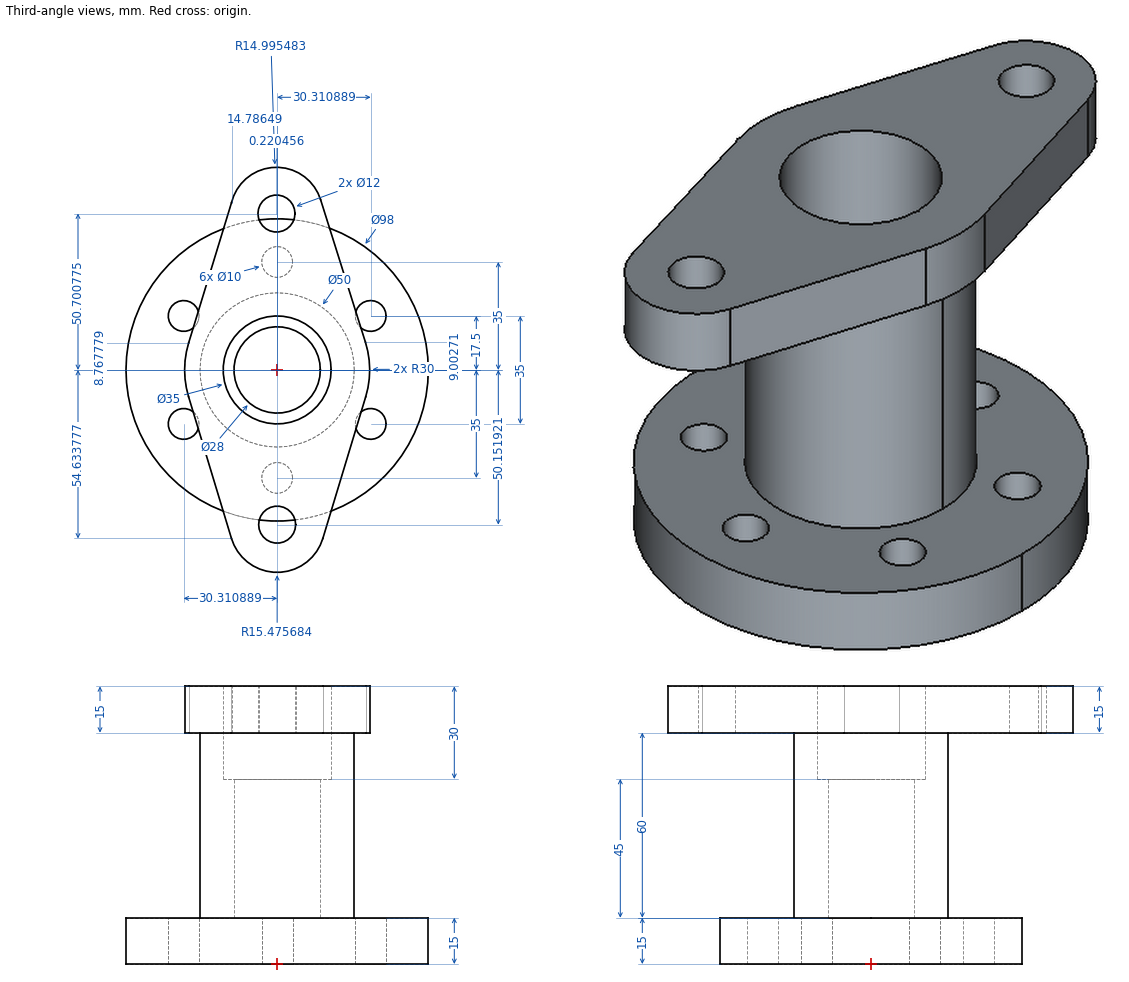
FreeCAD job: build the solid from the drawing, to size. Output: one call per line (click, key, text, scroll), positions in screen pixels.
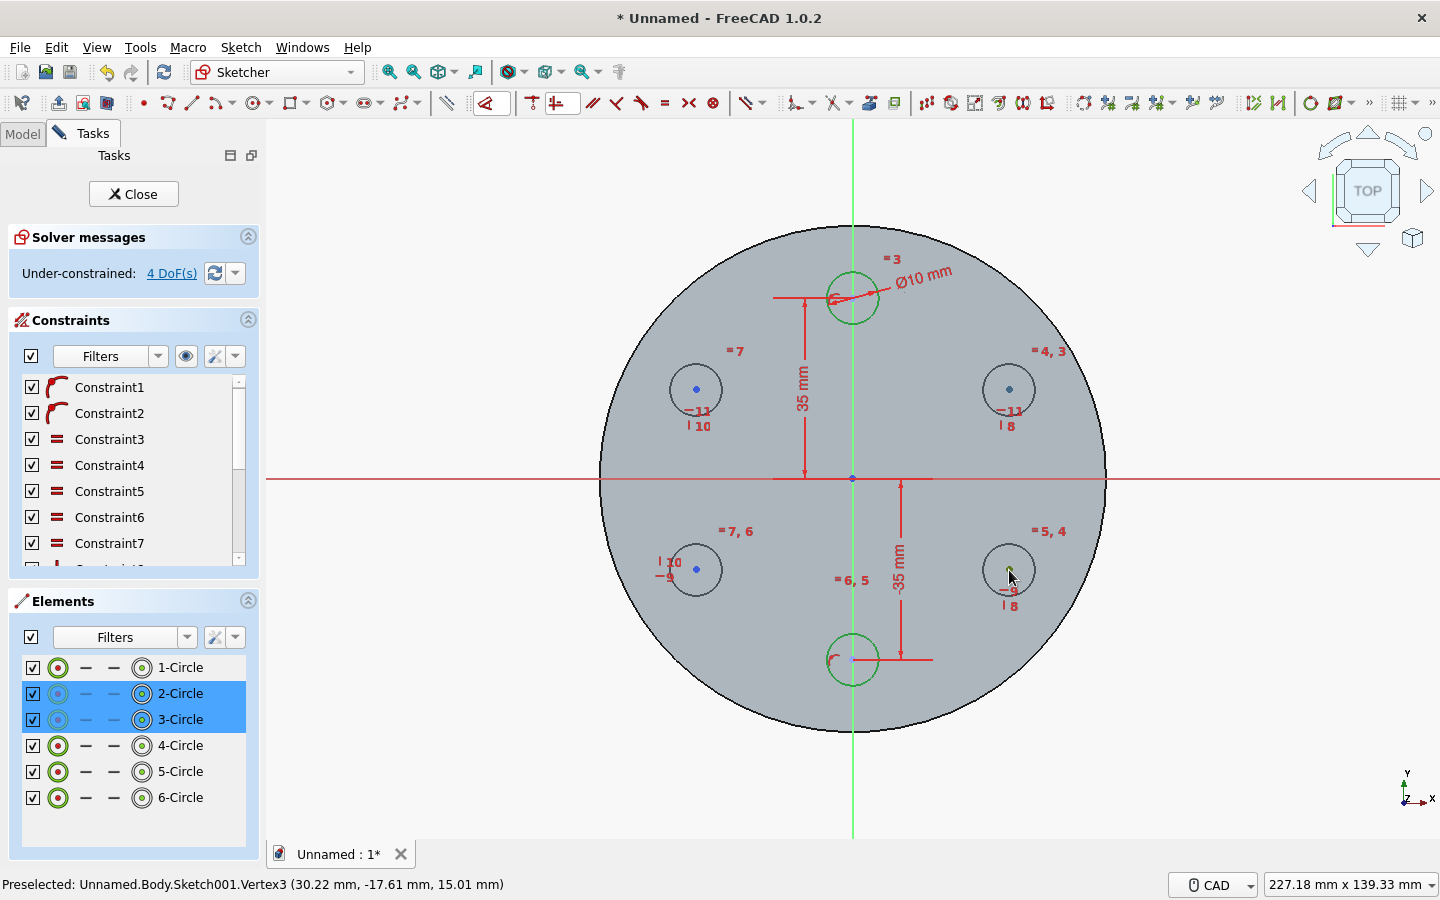
key(i)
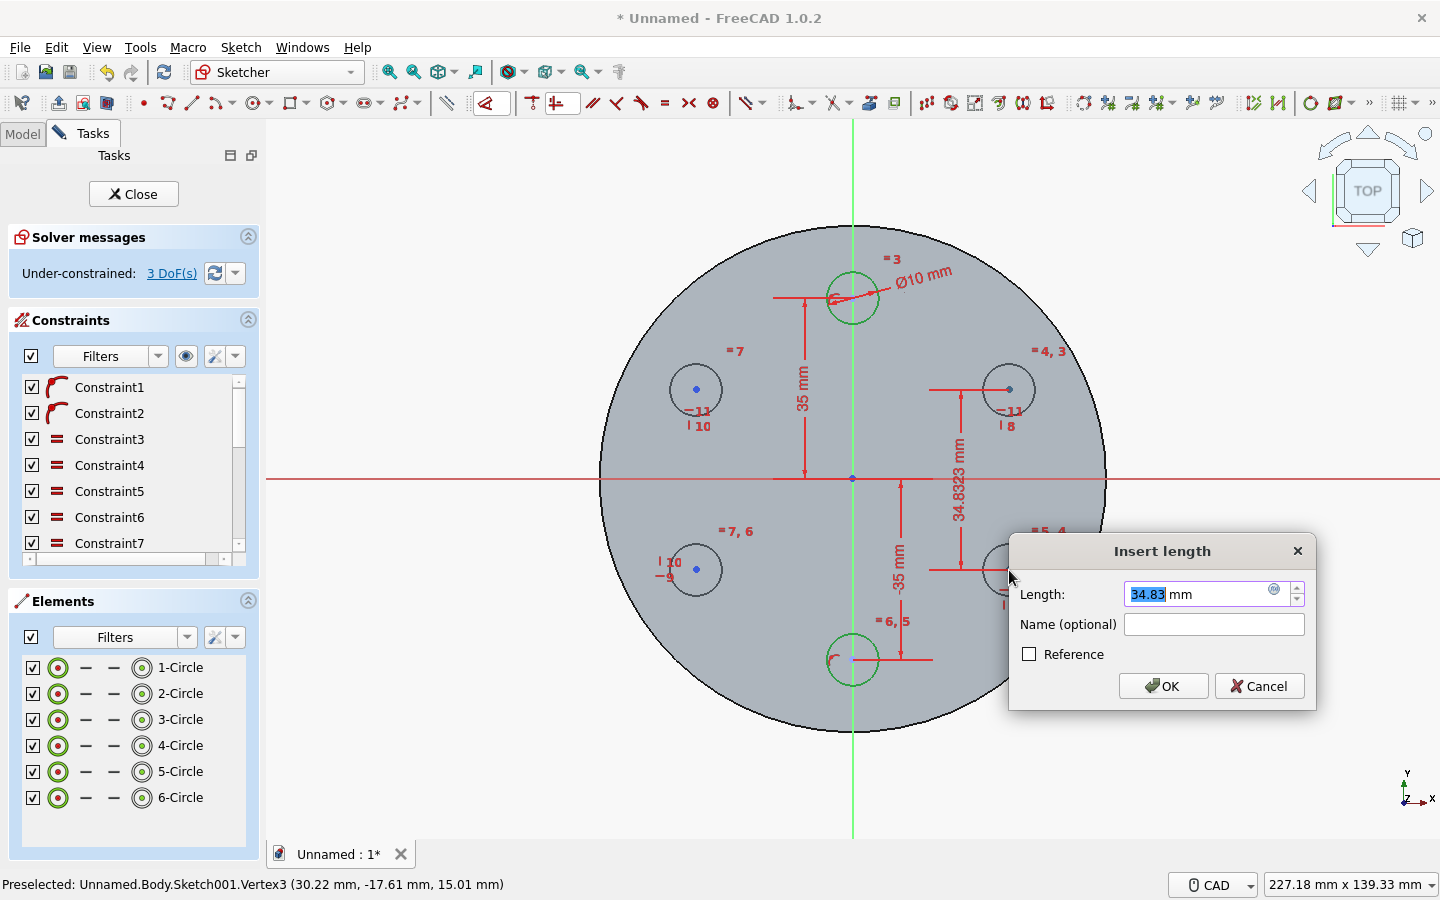
text(35)
key(Return)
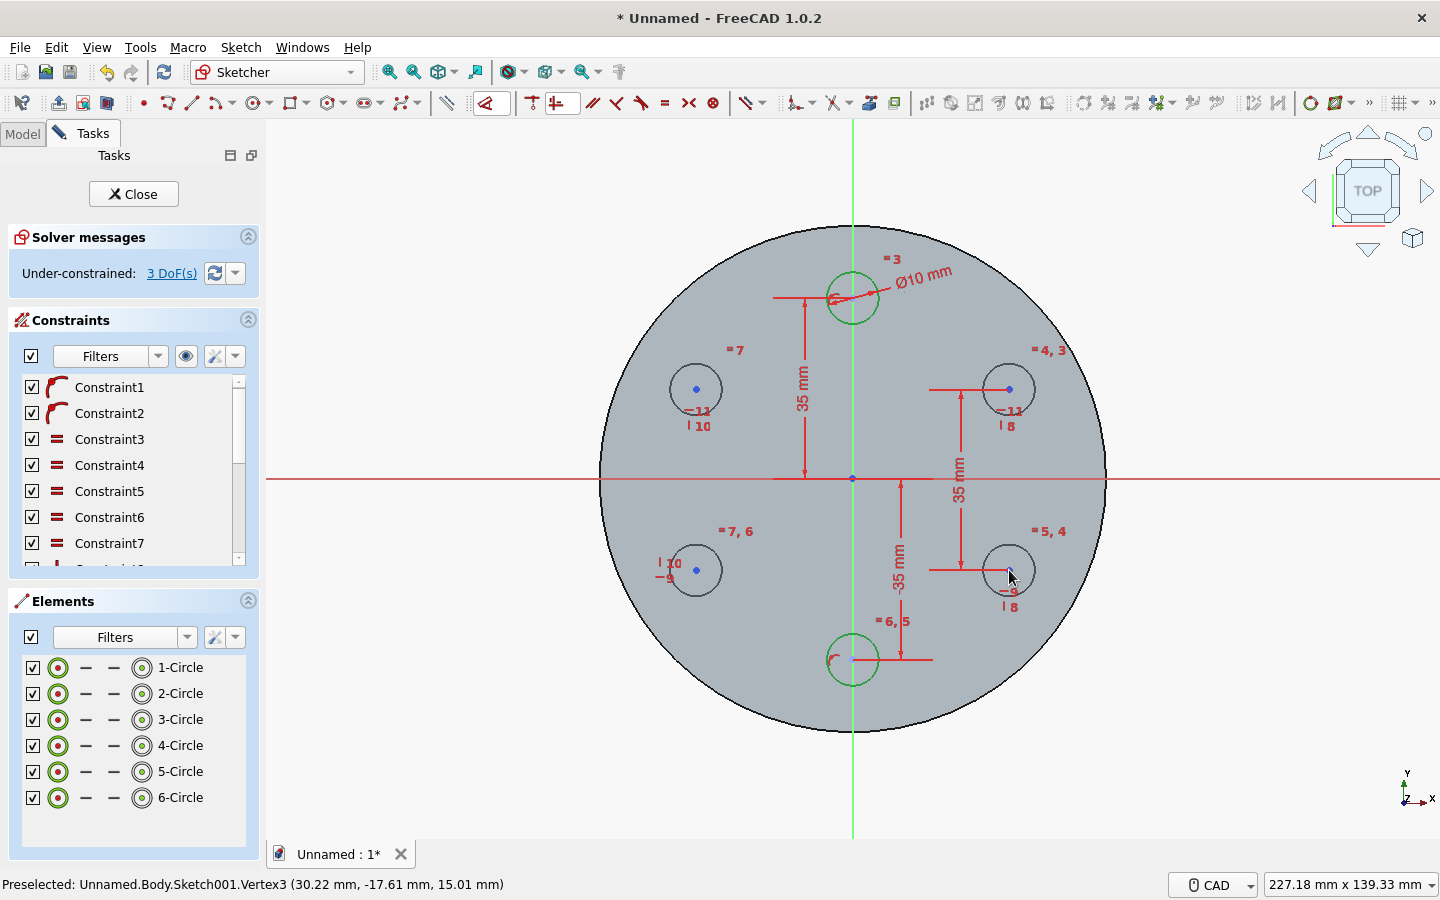
click(1009, 389)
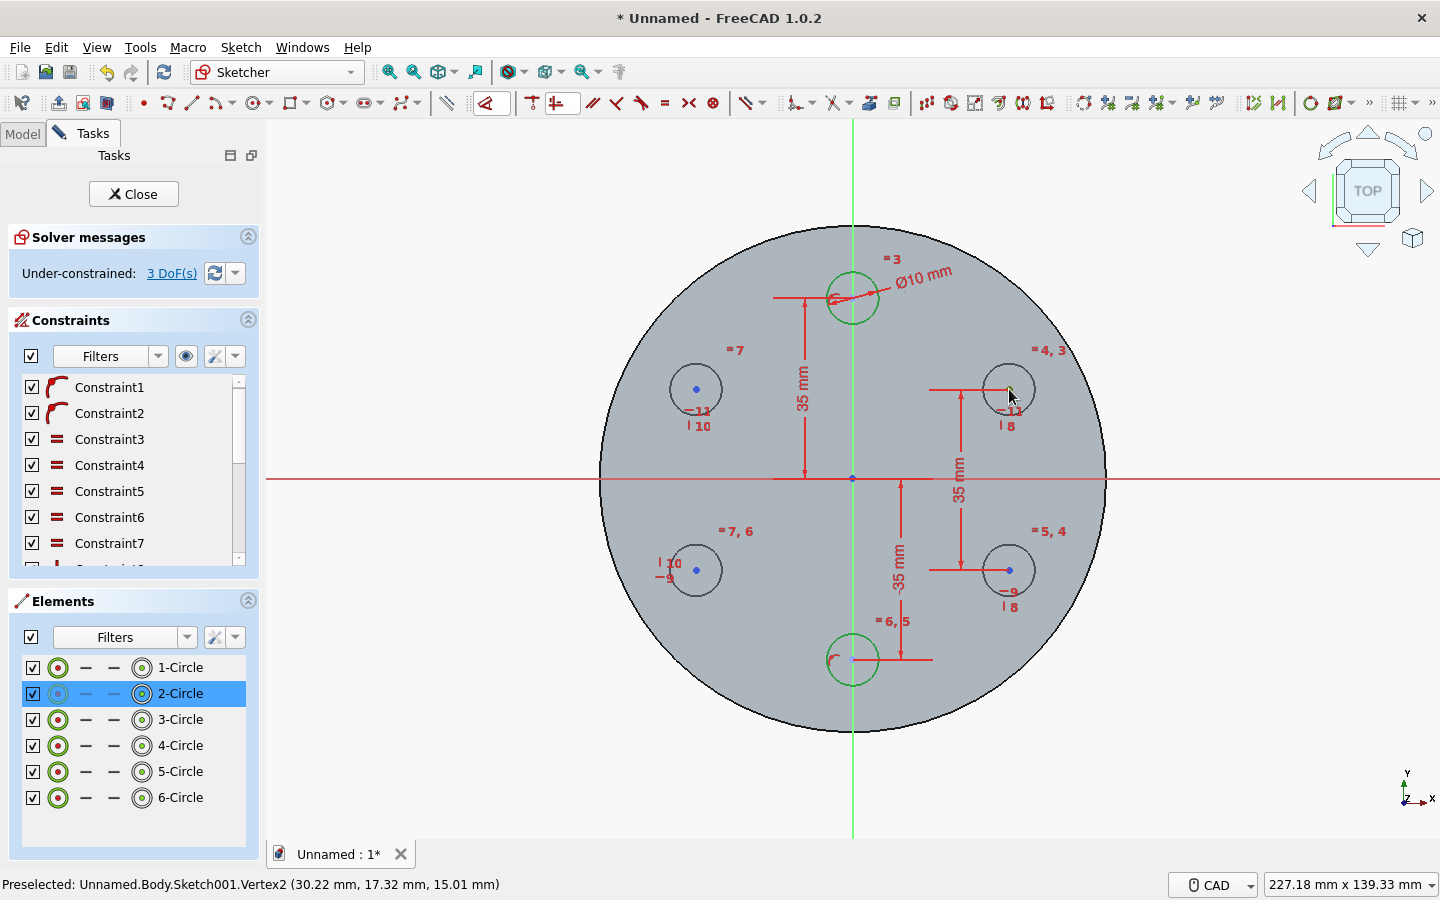
key(i)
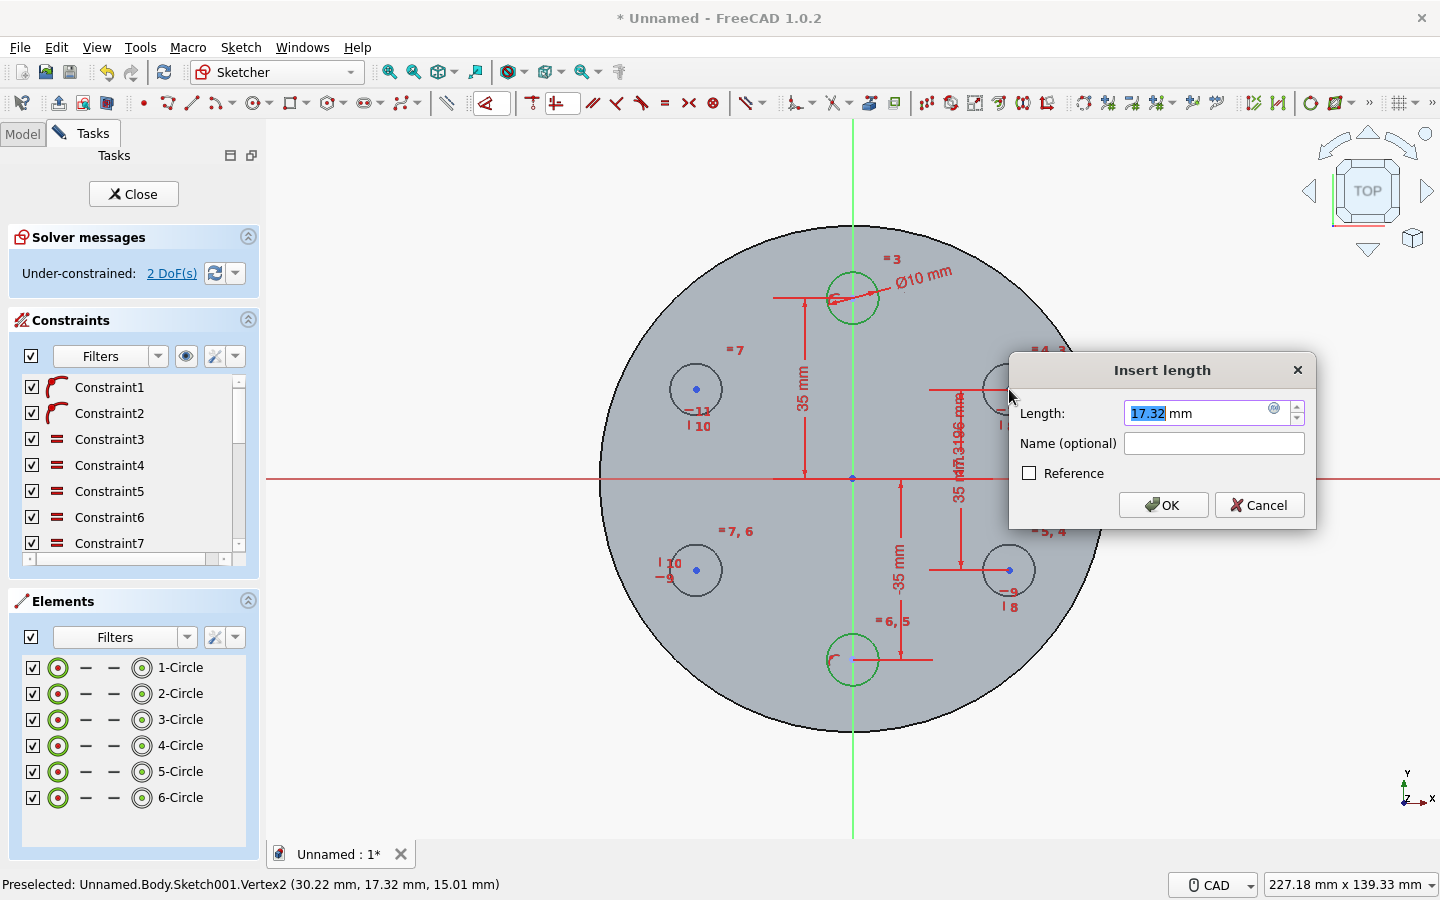
text(17.5)
key(Return)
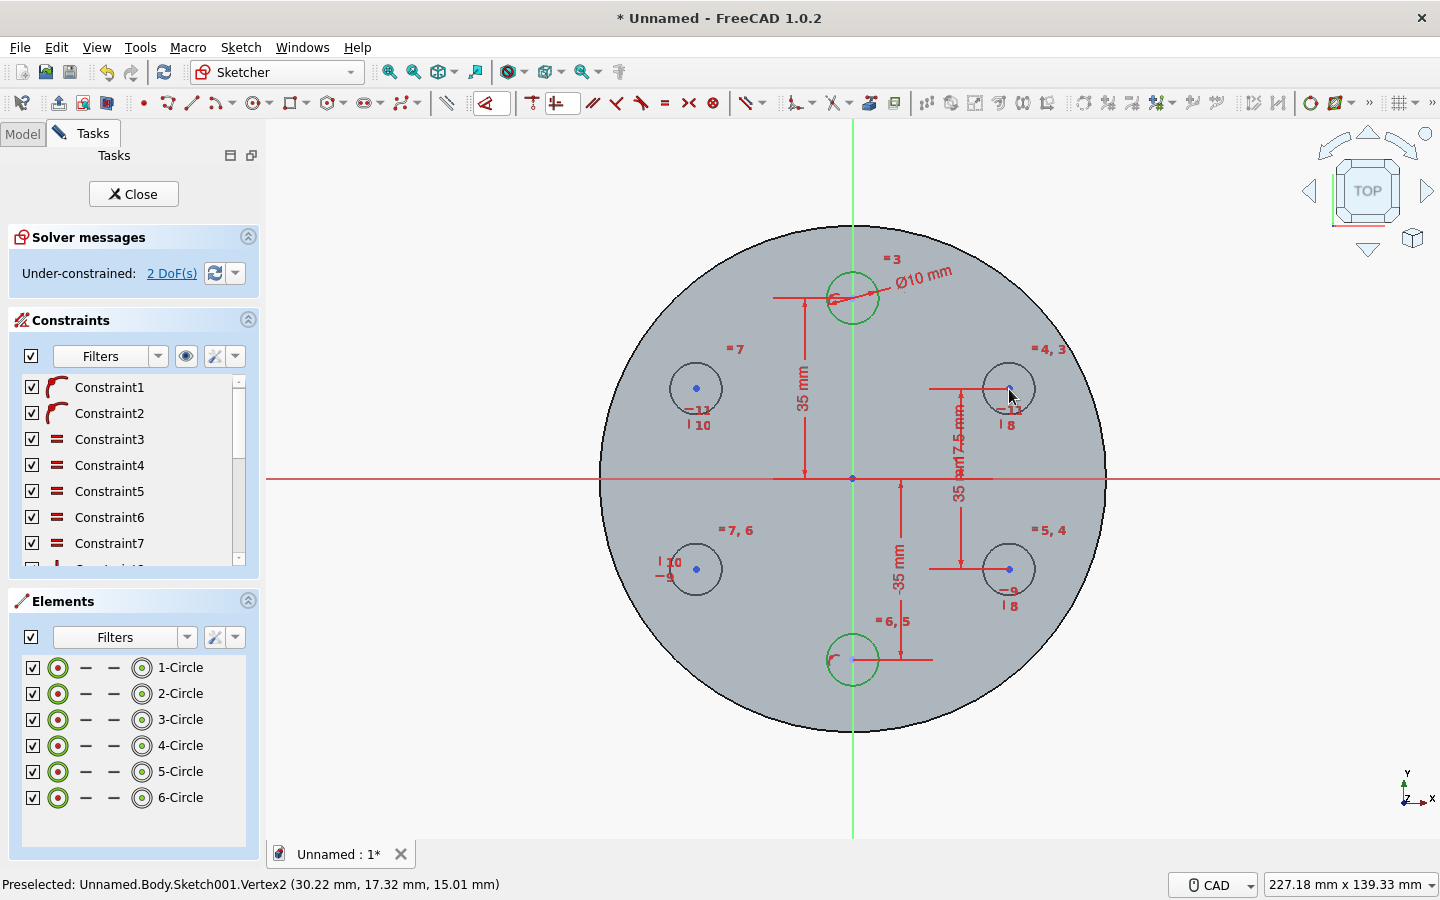
click(1009, 389)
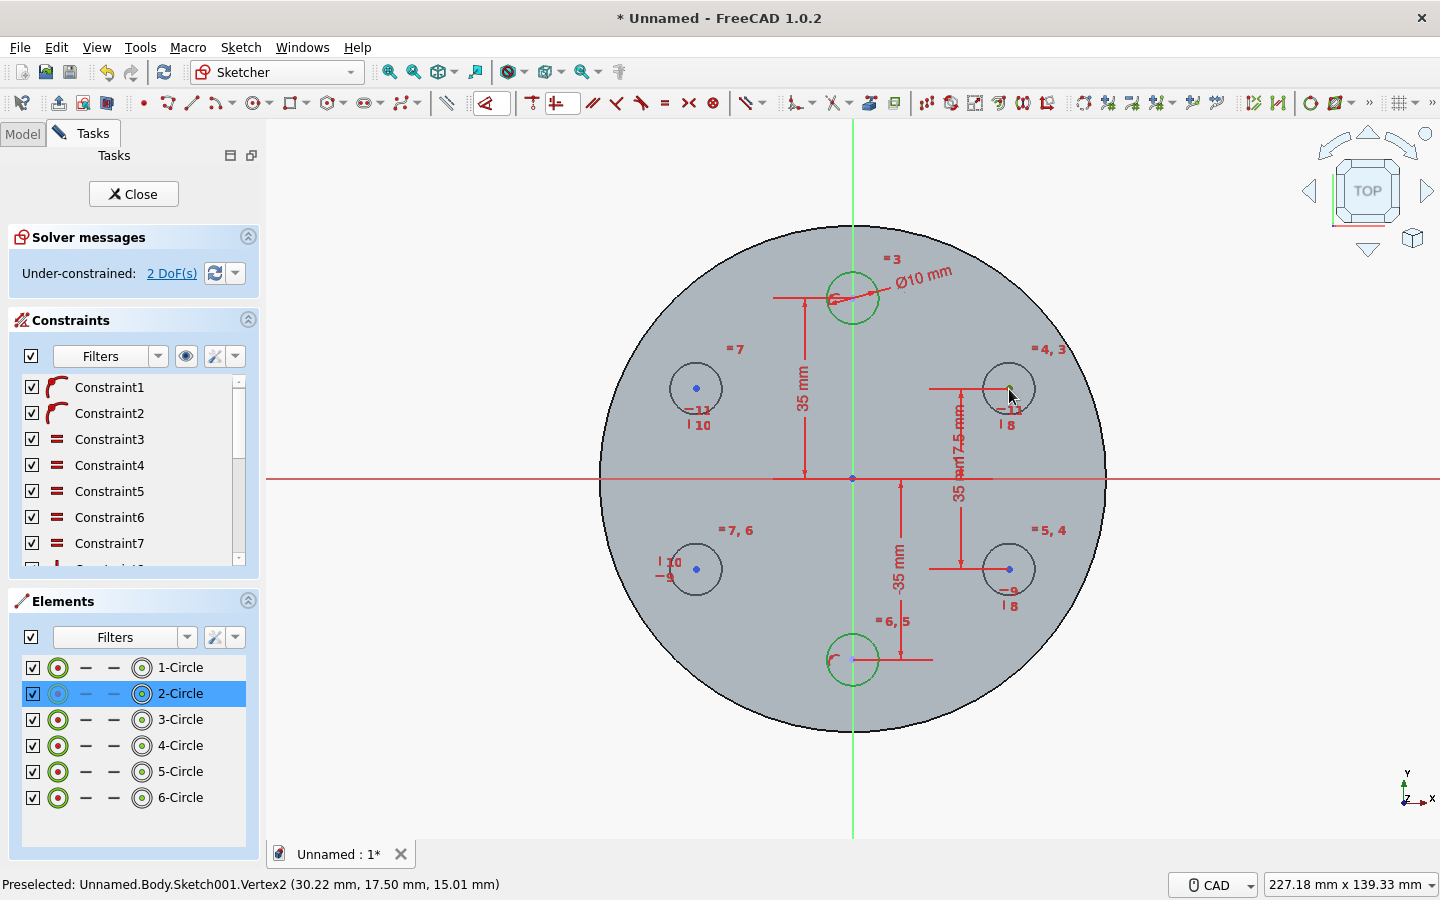
key(l)